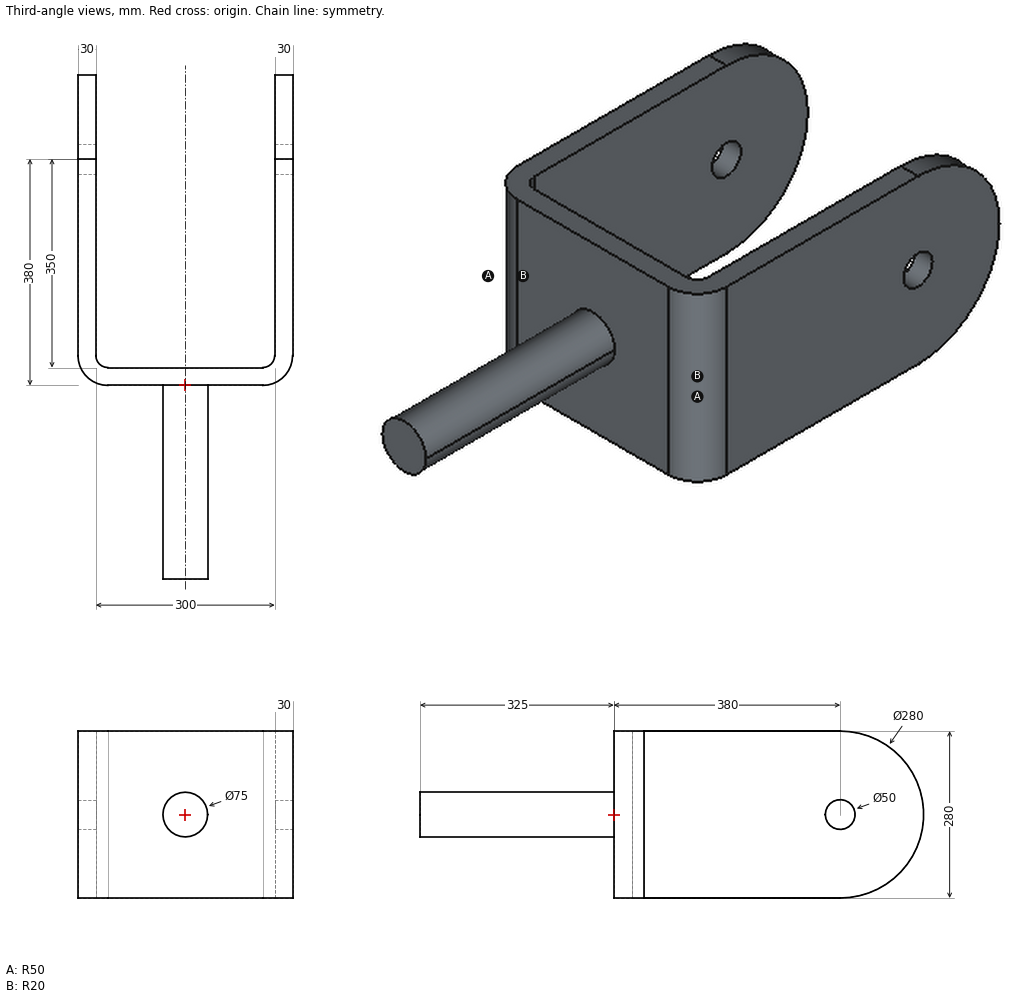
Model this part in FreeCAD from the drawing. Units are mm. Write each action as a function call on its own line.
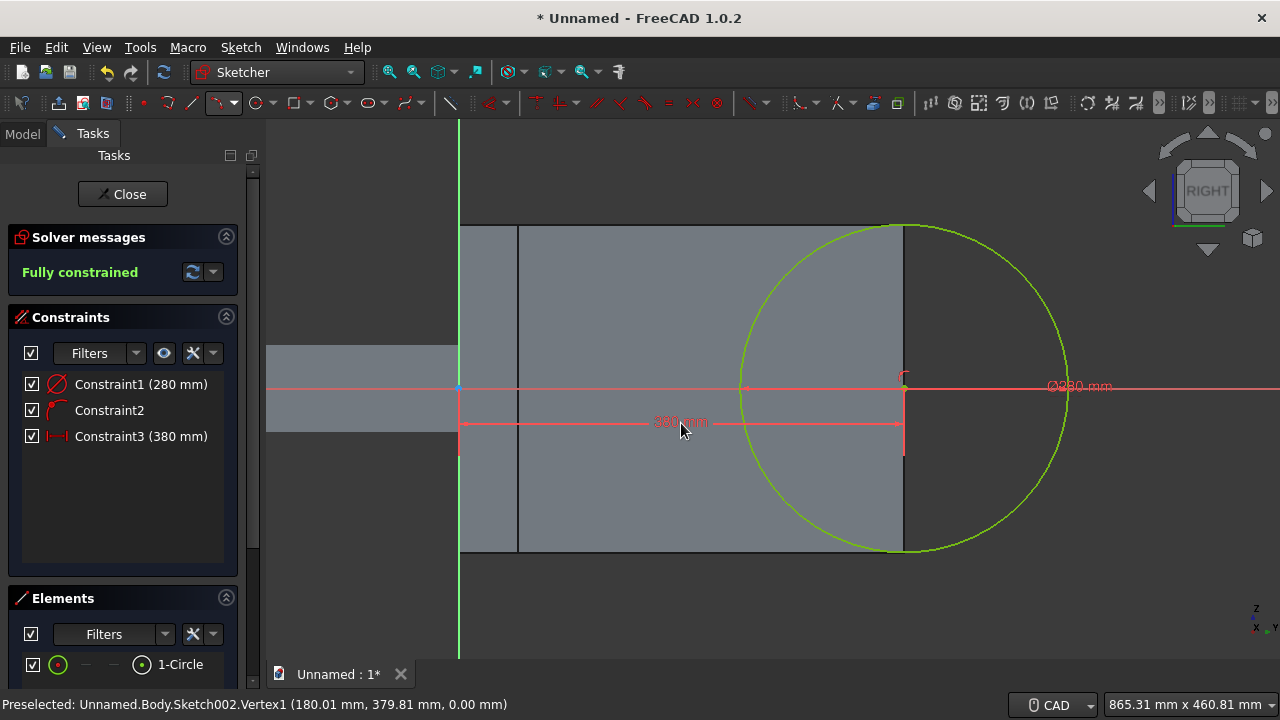
click(123, 194)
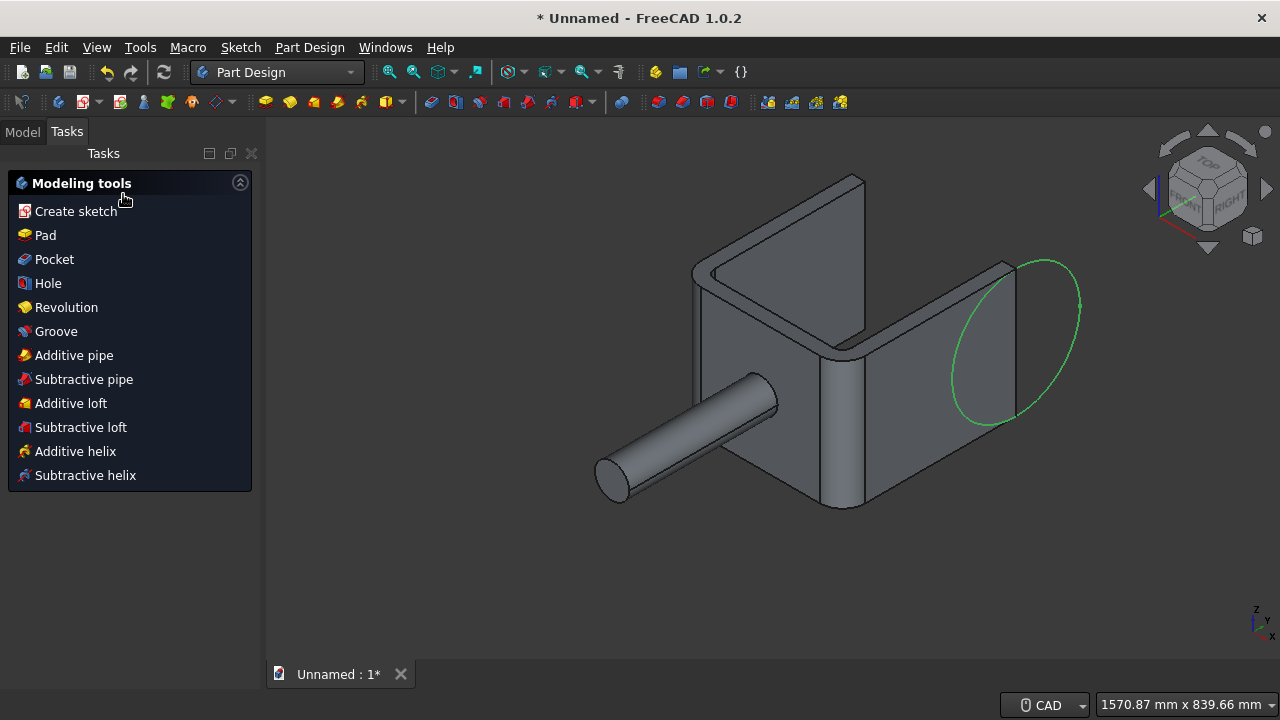
click(266, 102)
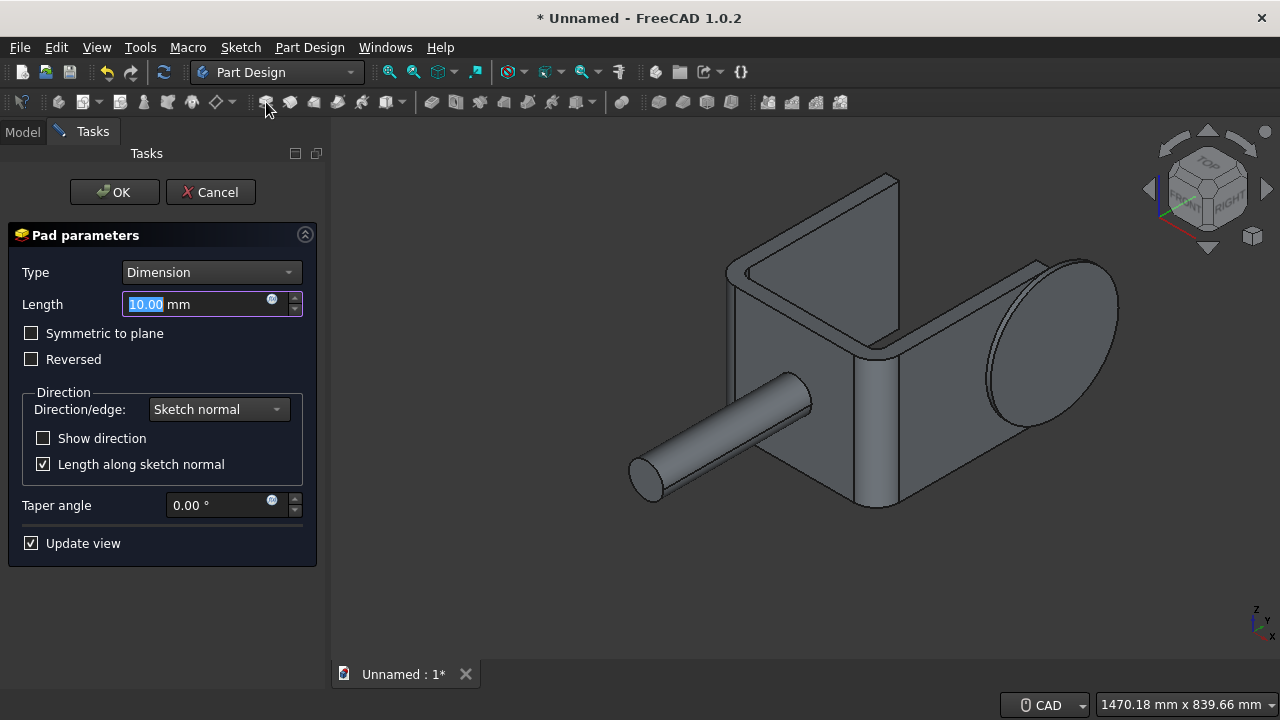
text(30)
key(Tab)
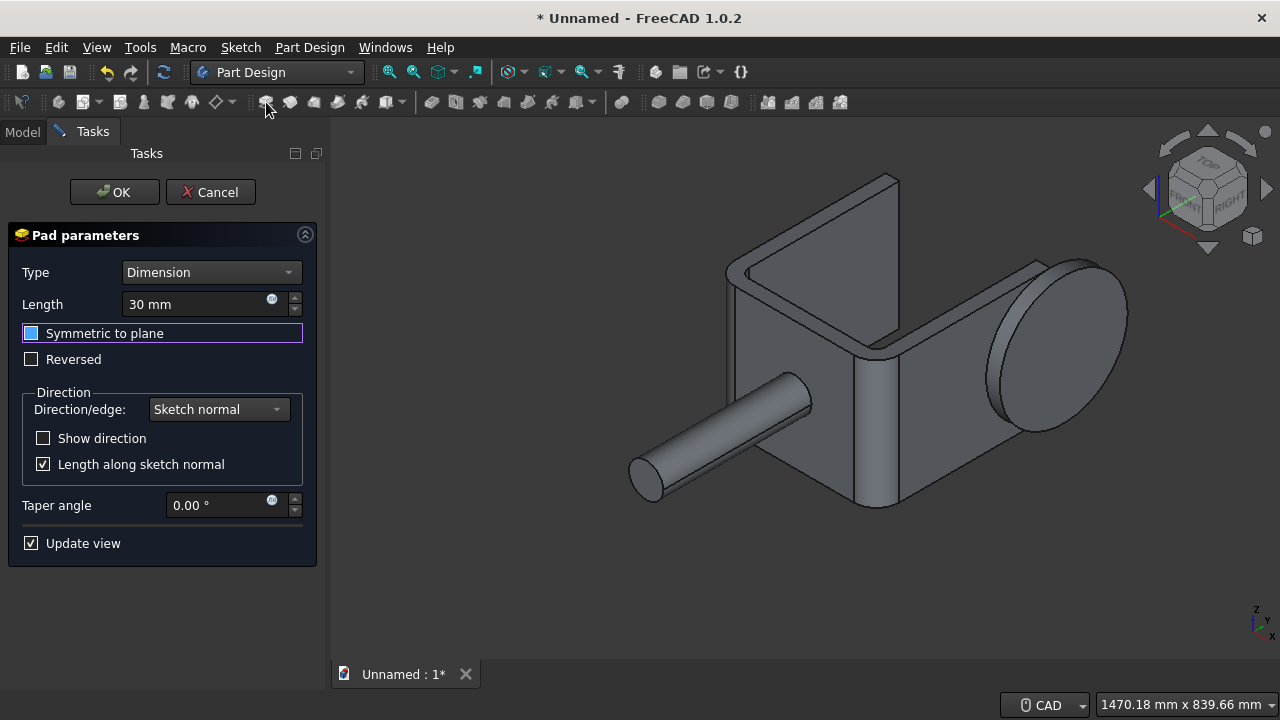
click(30, 359)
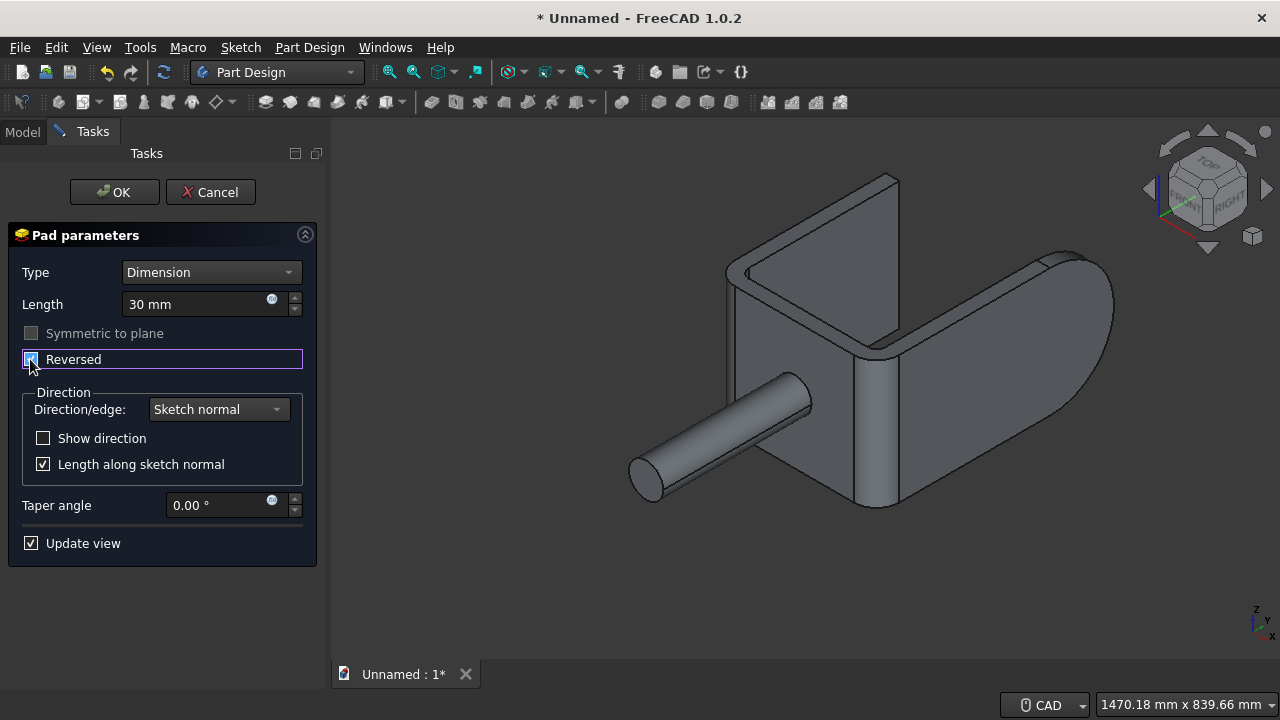
click(115, 192)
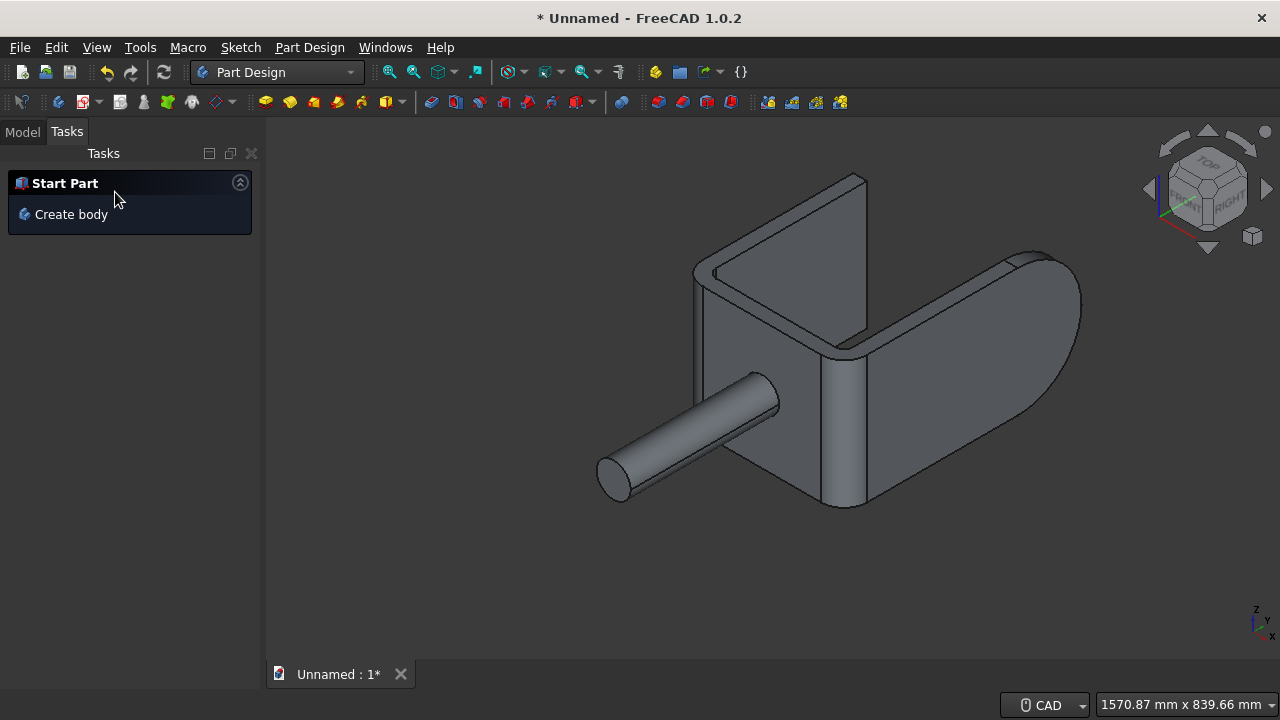
click(23, 131)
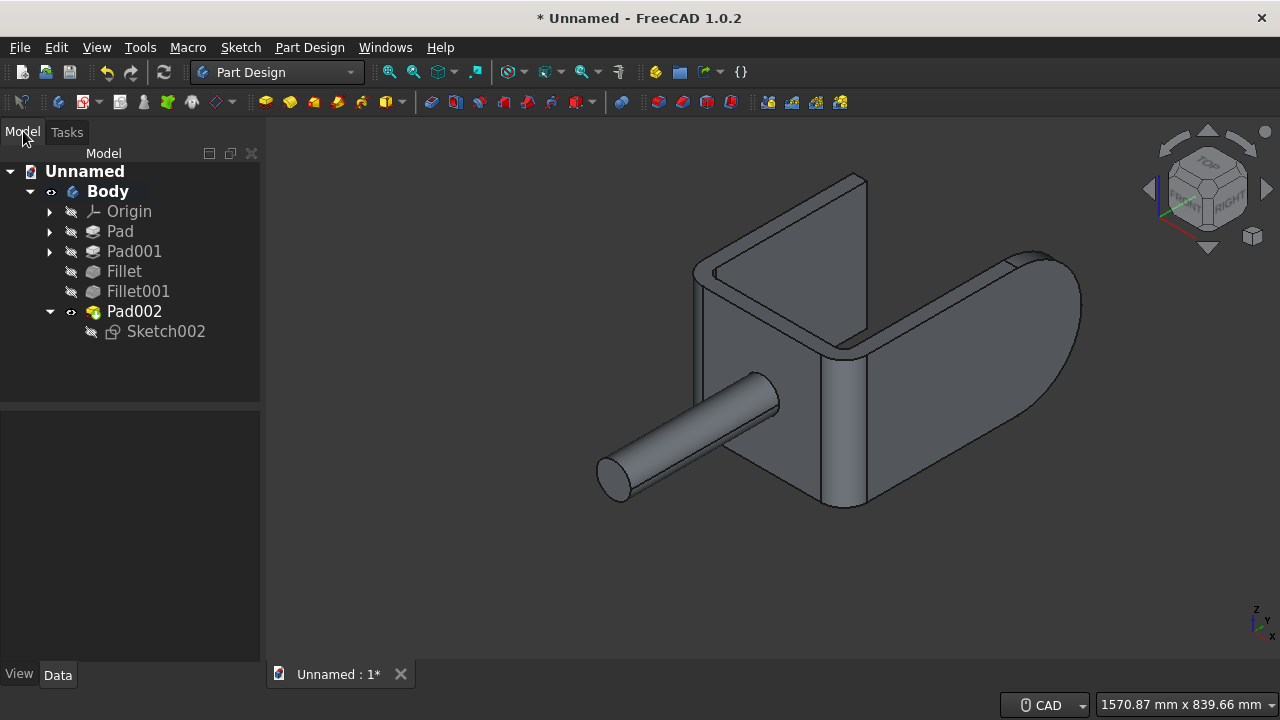
click(116, 312)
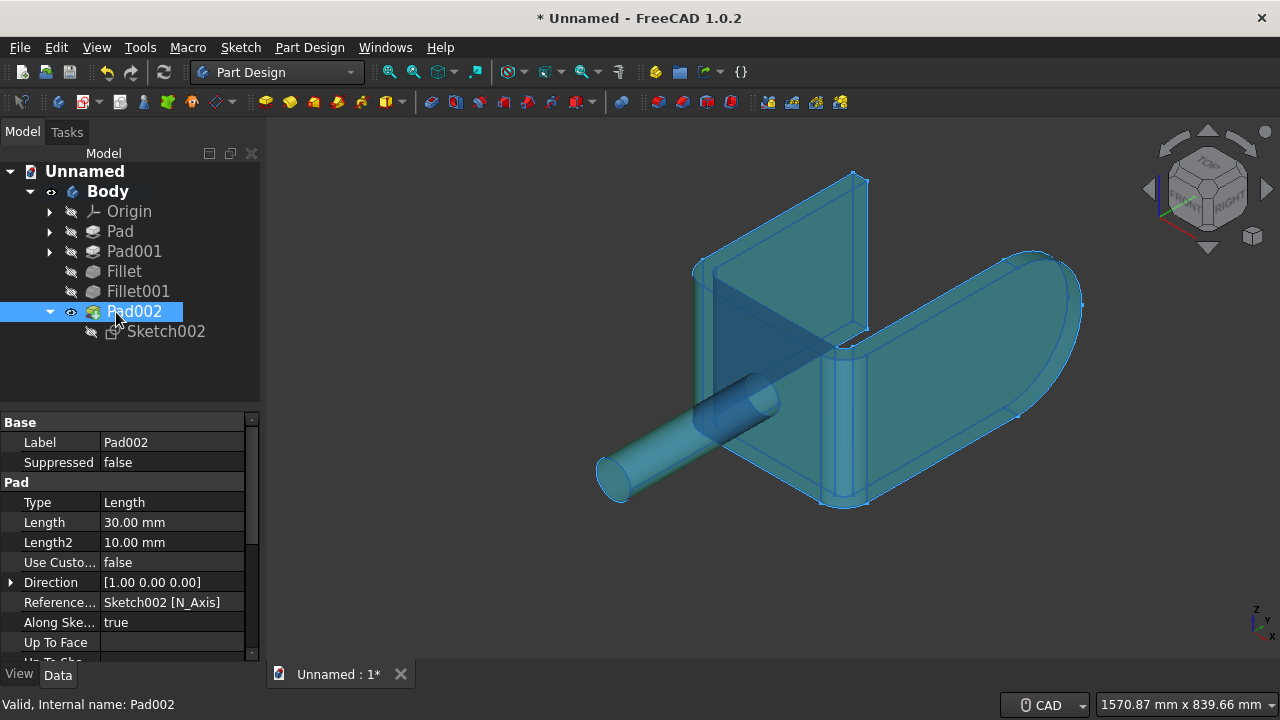
click(768, 102)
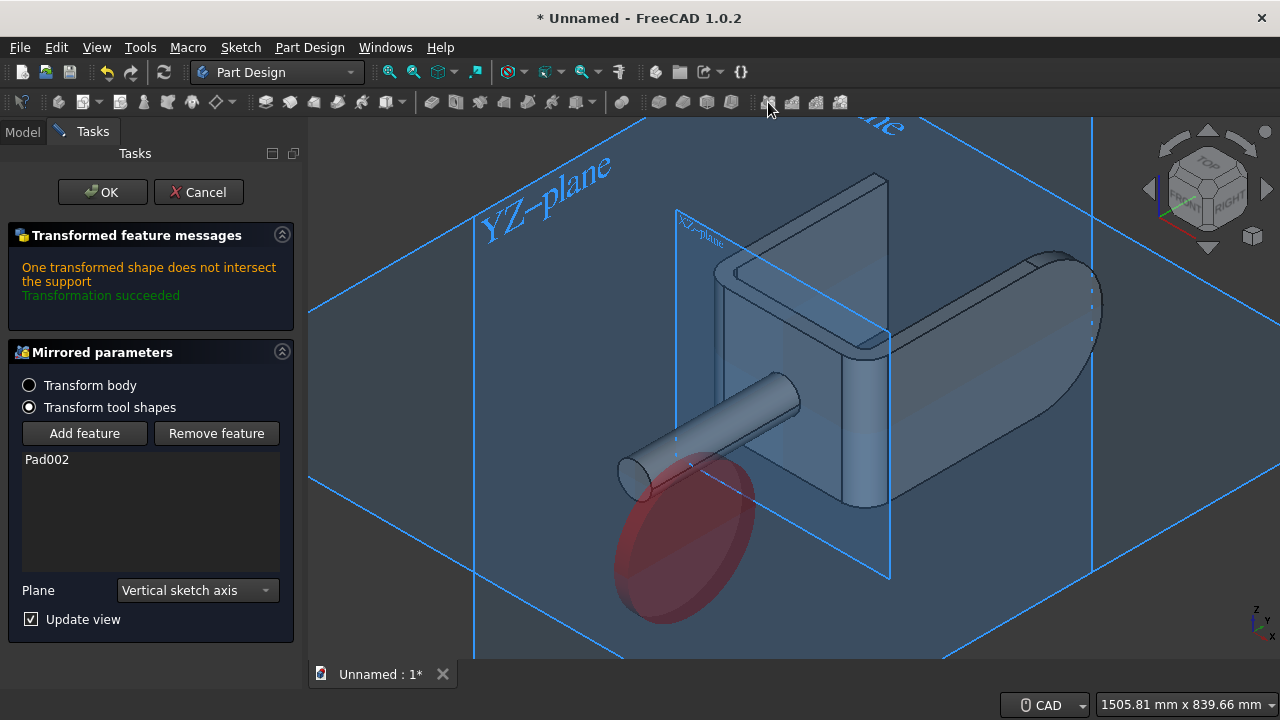
click(198, 590)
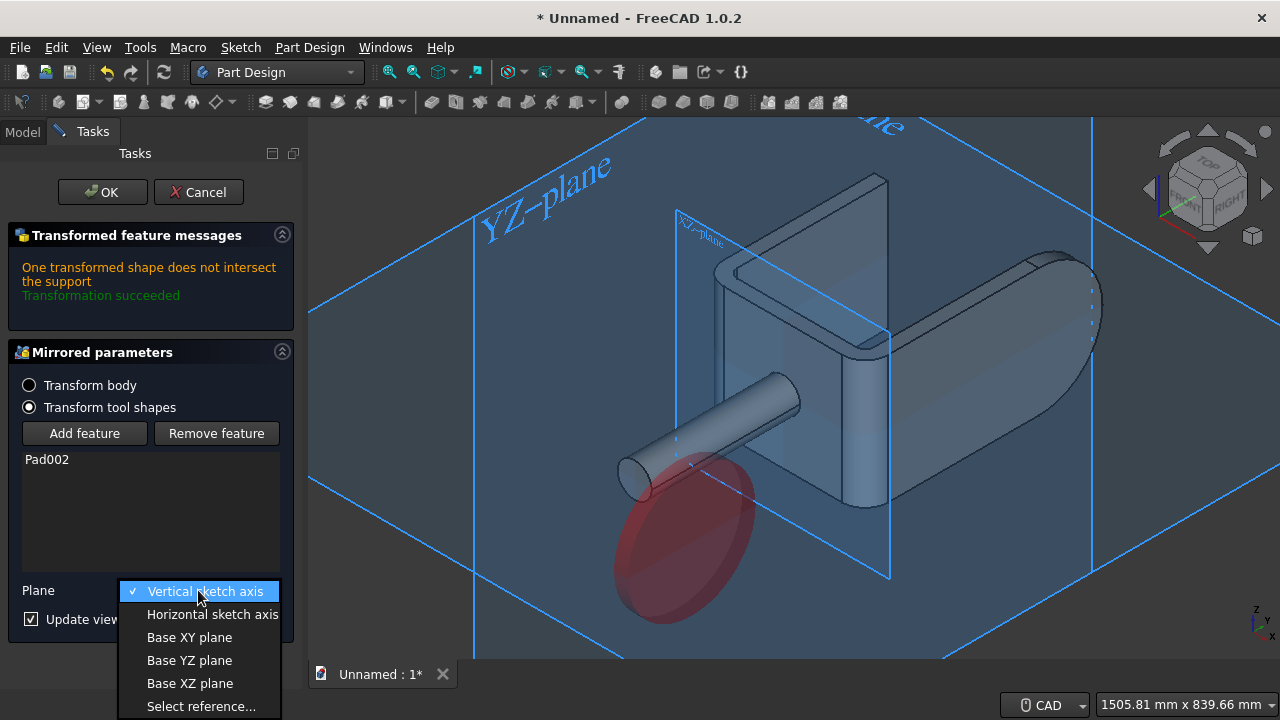
click(198, 660)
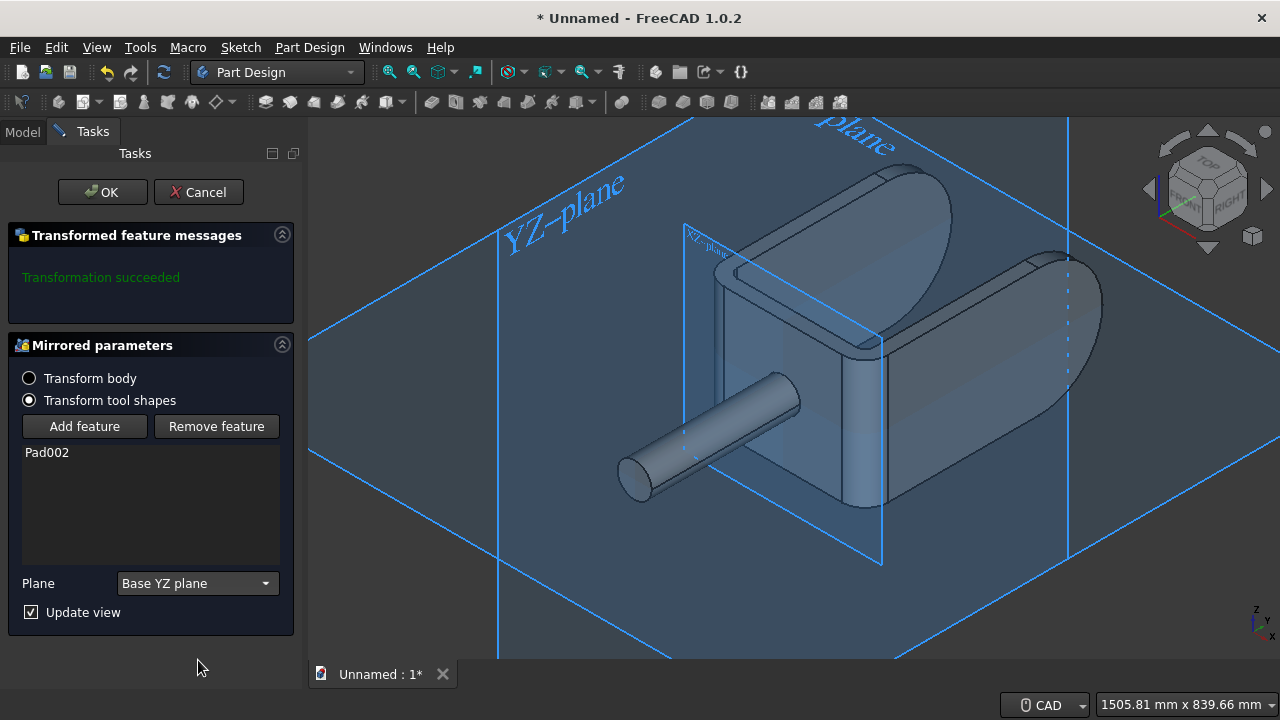
click(103, 192)